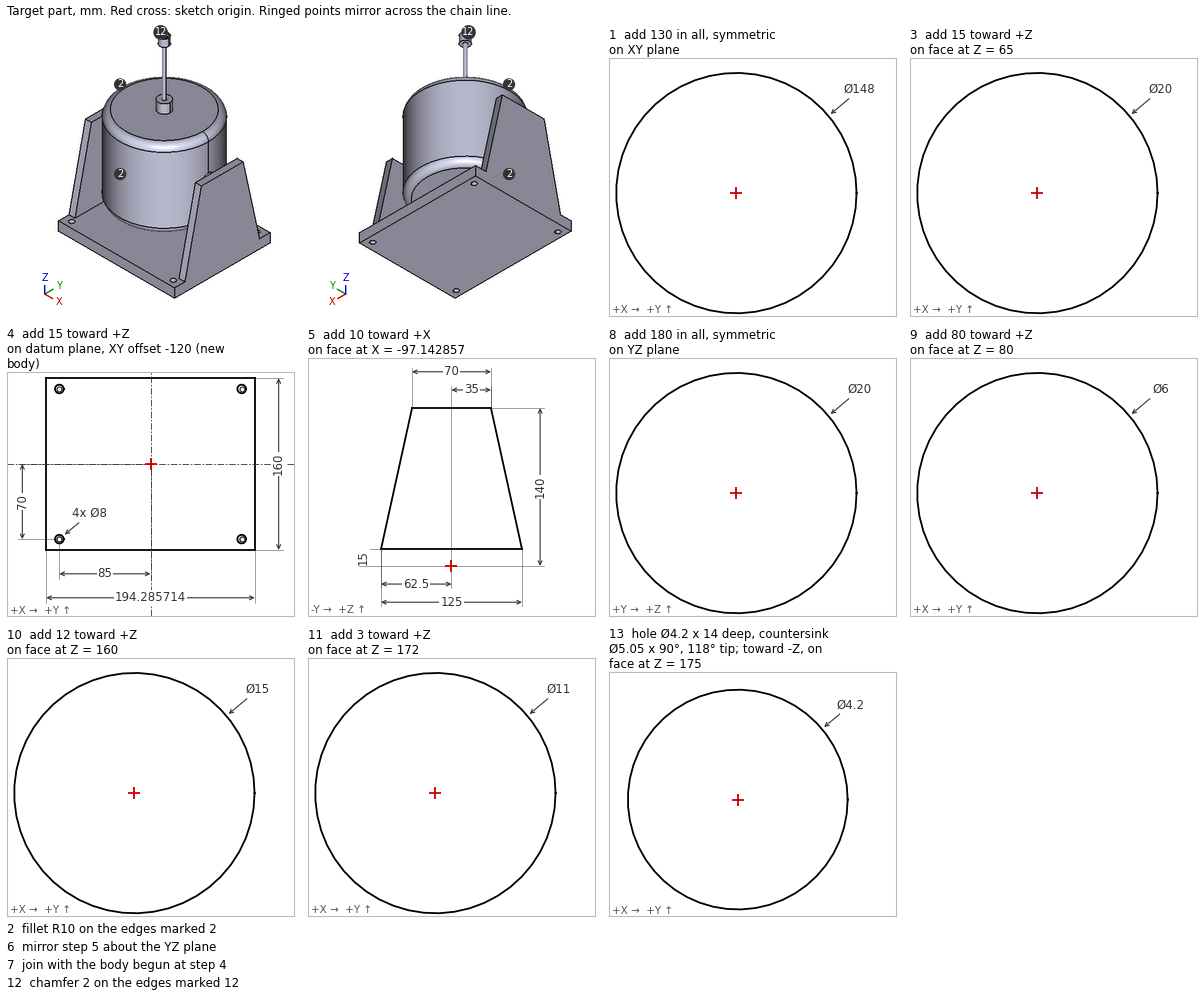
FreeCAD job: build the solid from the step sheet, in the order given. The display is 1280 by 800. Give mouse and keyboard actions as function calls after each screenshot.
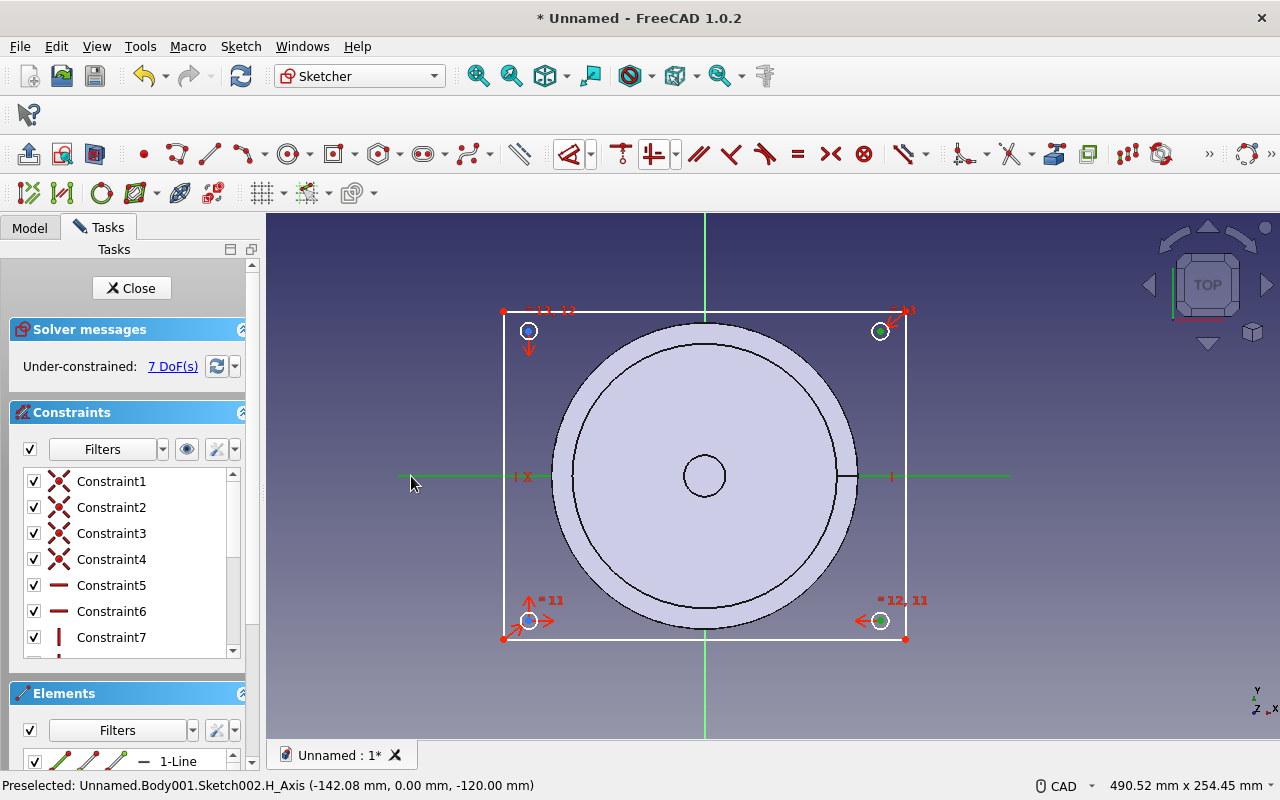
key(s)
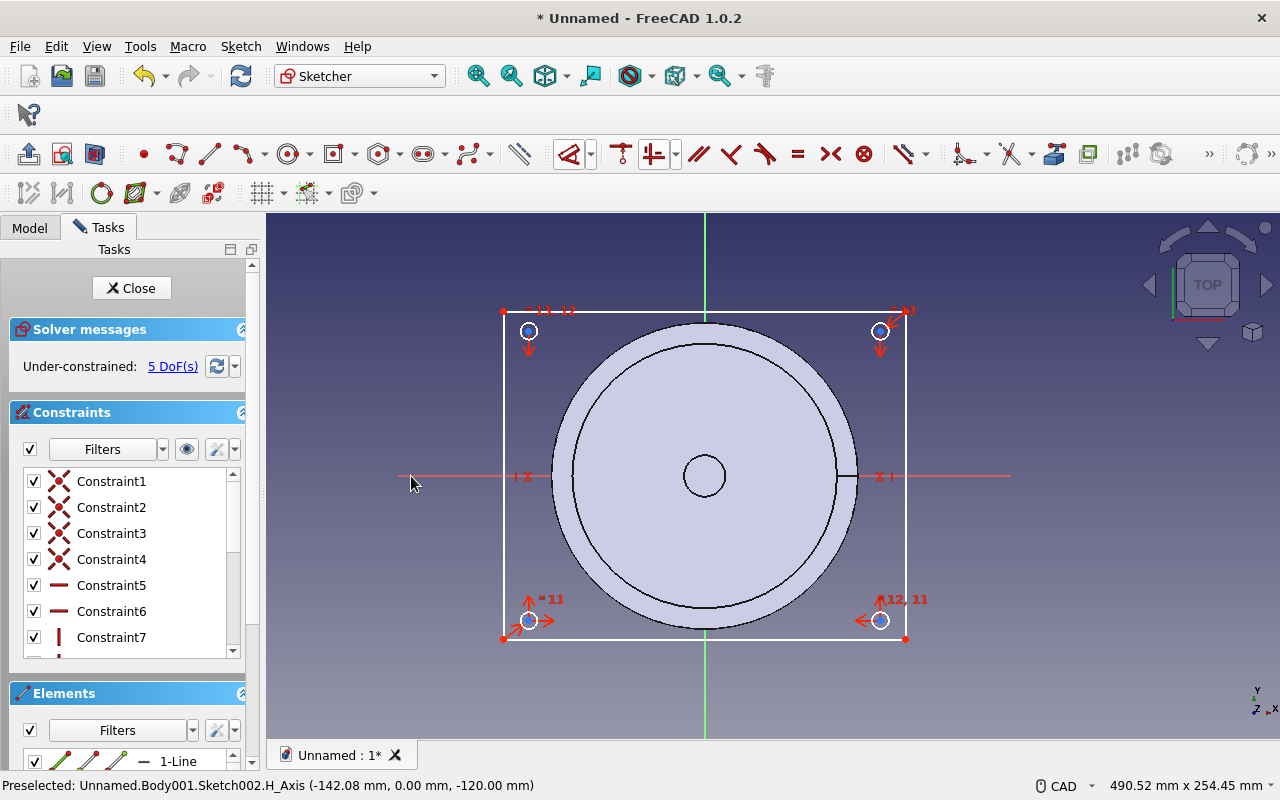
scroll(529, 629, up, 5)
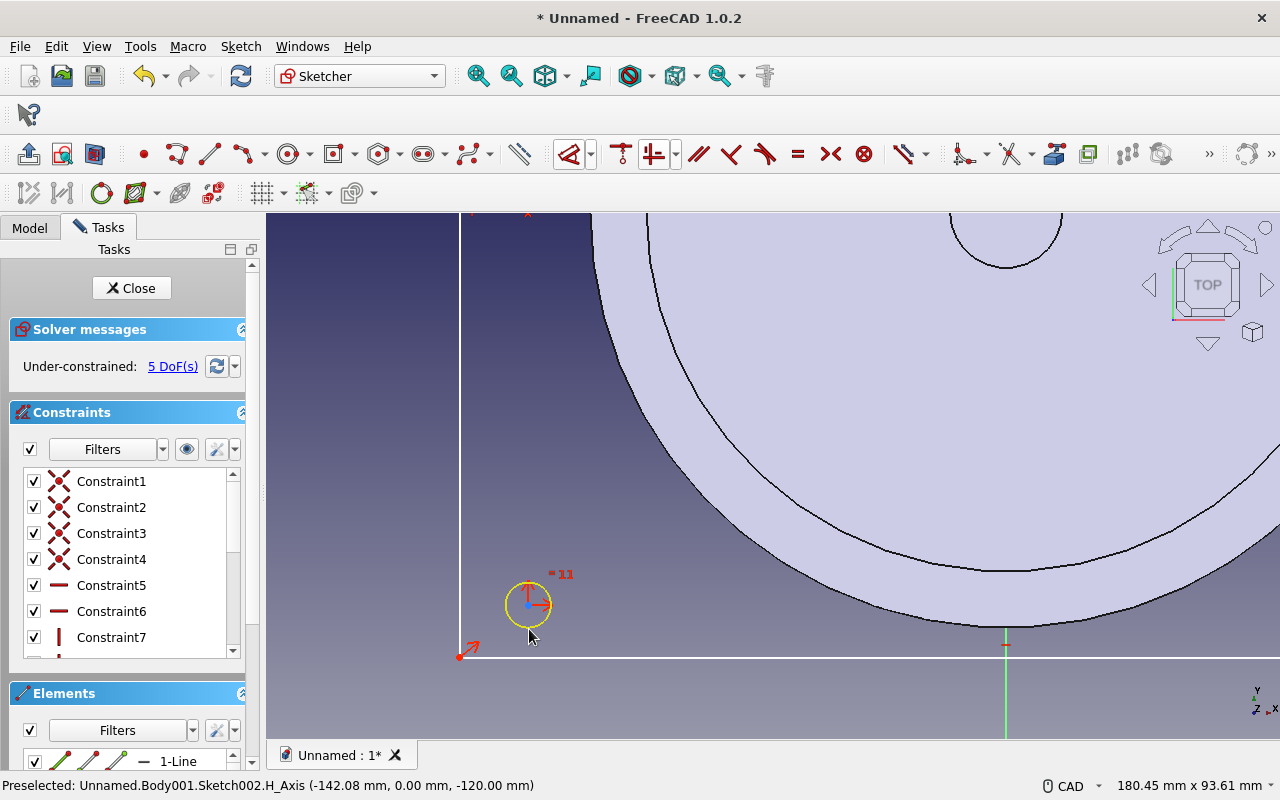
click(528, 628)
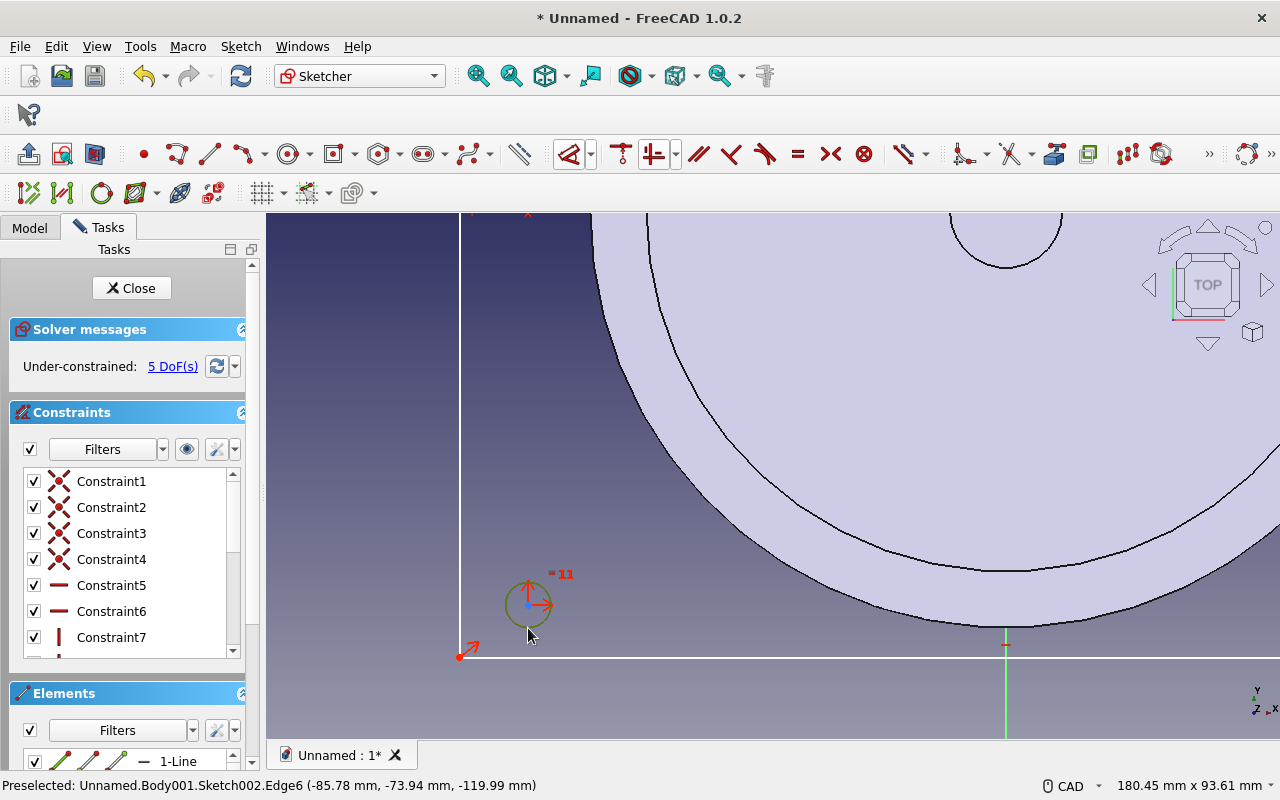
key(k)
key(o)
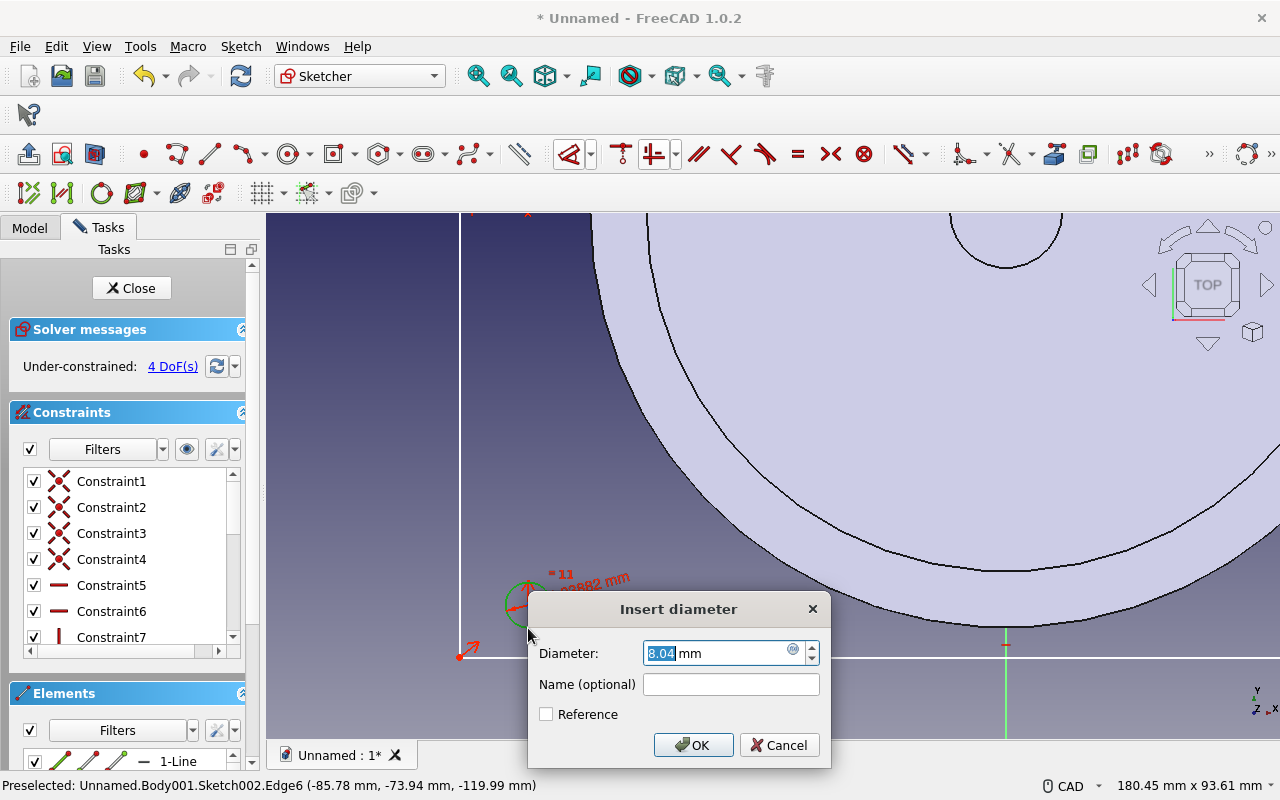
text(8)
key(Return)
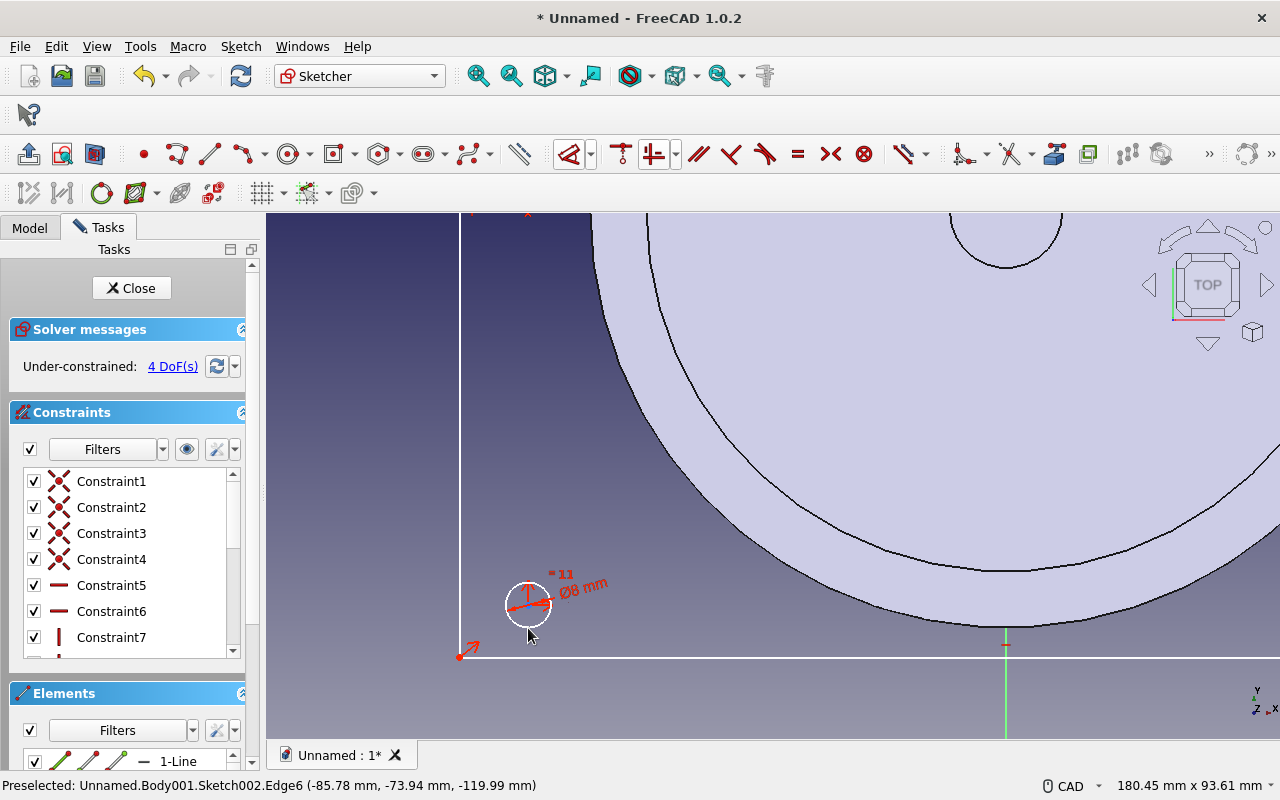
click(528, 605)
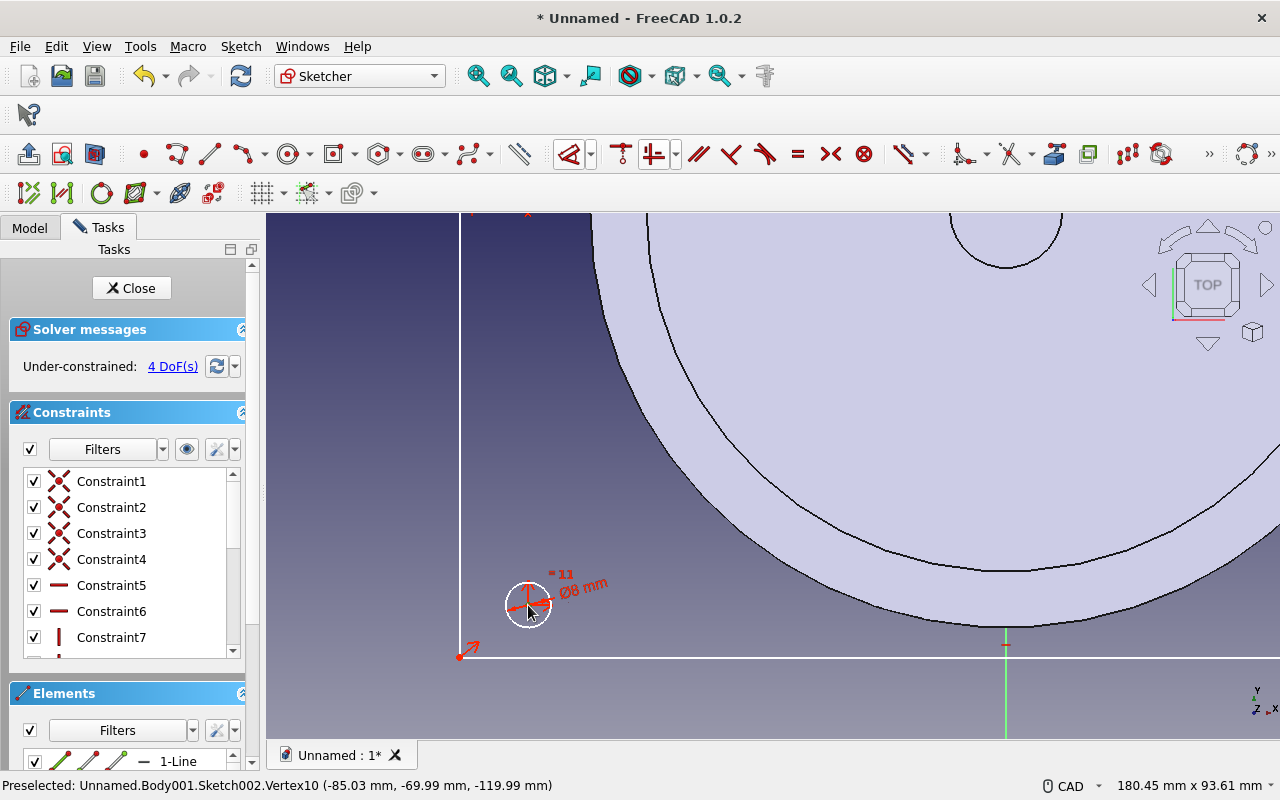
click(590, 154)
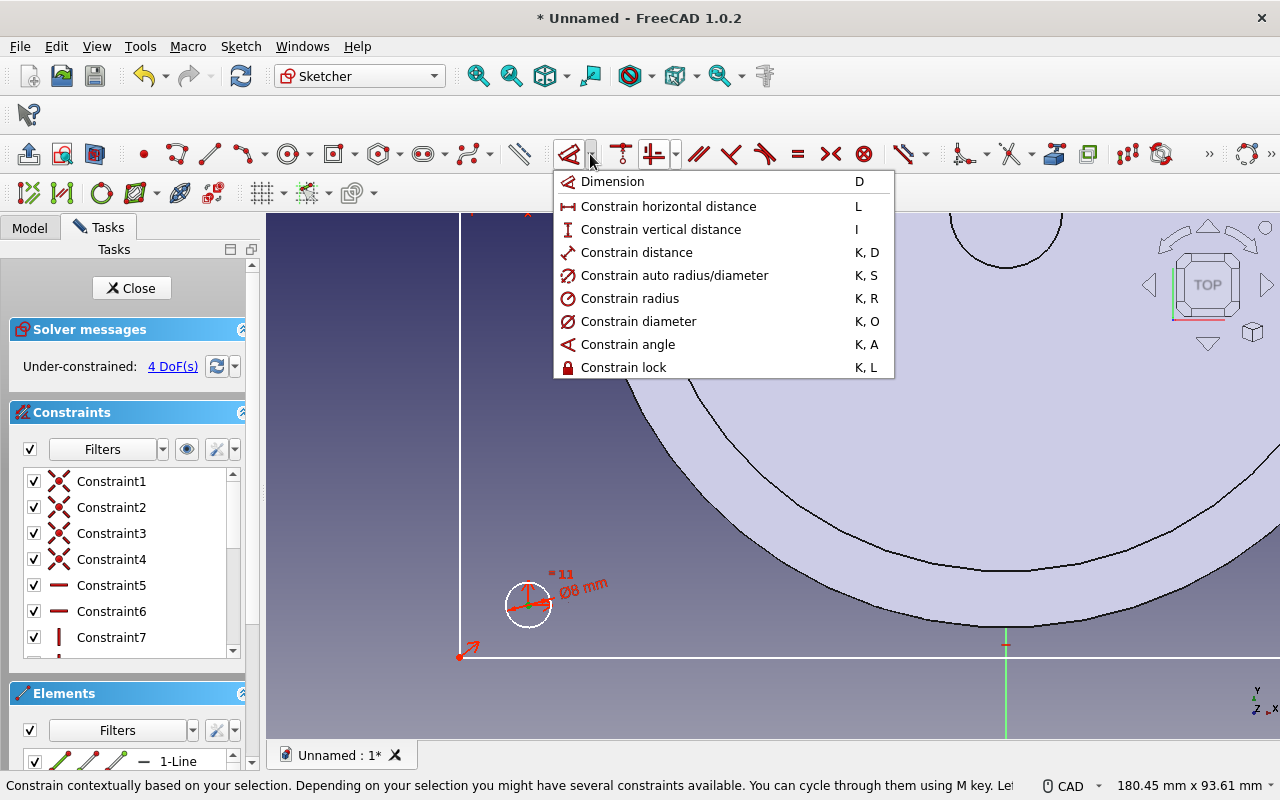
click(724, 206)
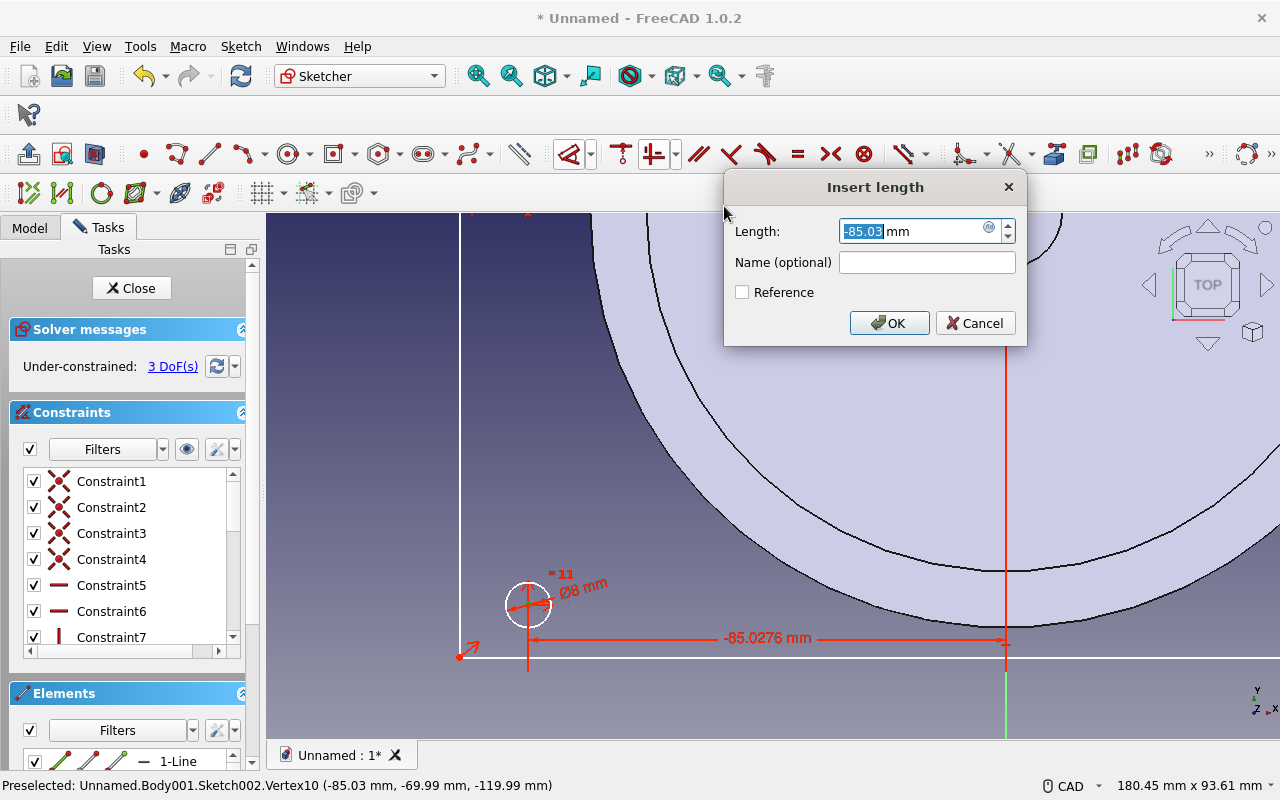
text(-85)
key(Return)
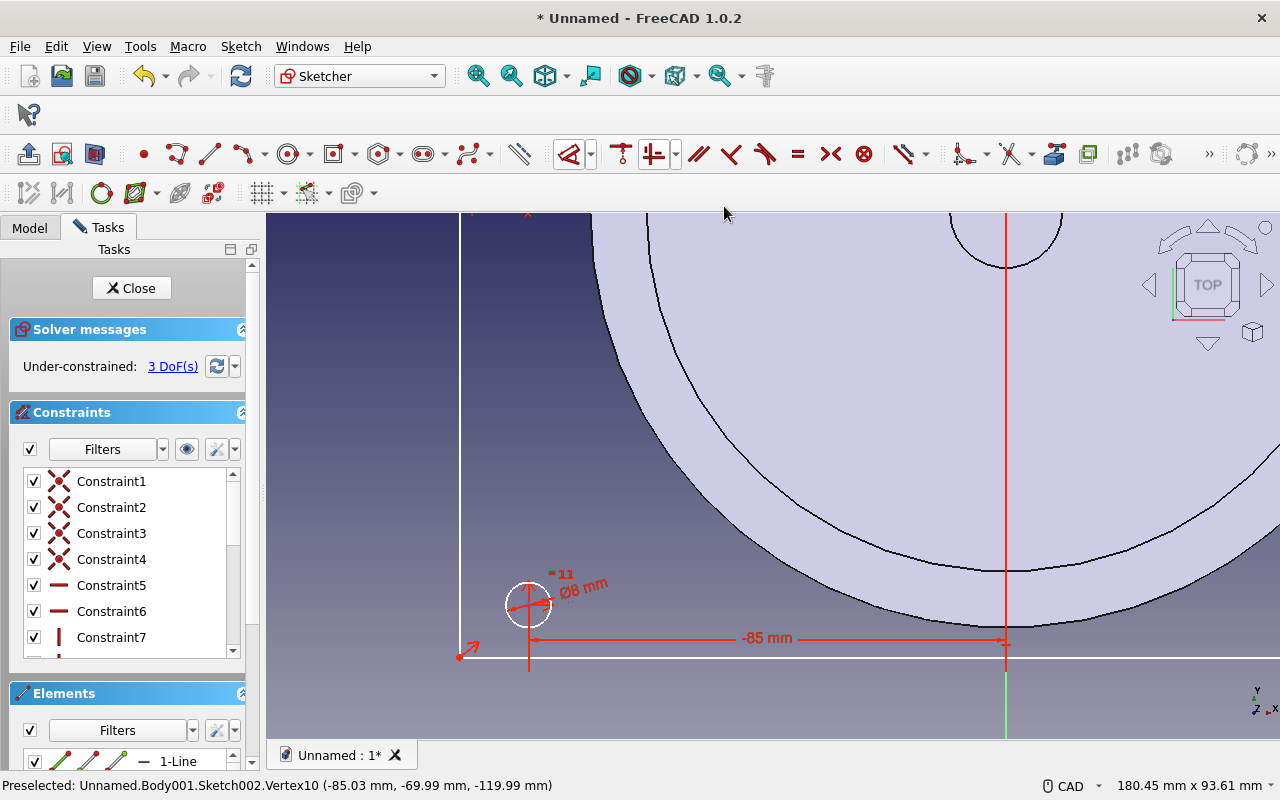
click(529, 605)